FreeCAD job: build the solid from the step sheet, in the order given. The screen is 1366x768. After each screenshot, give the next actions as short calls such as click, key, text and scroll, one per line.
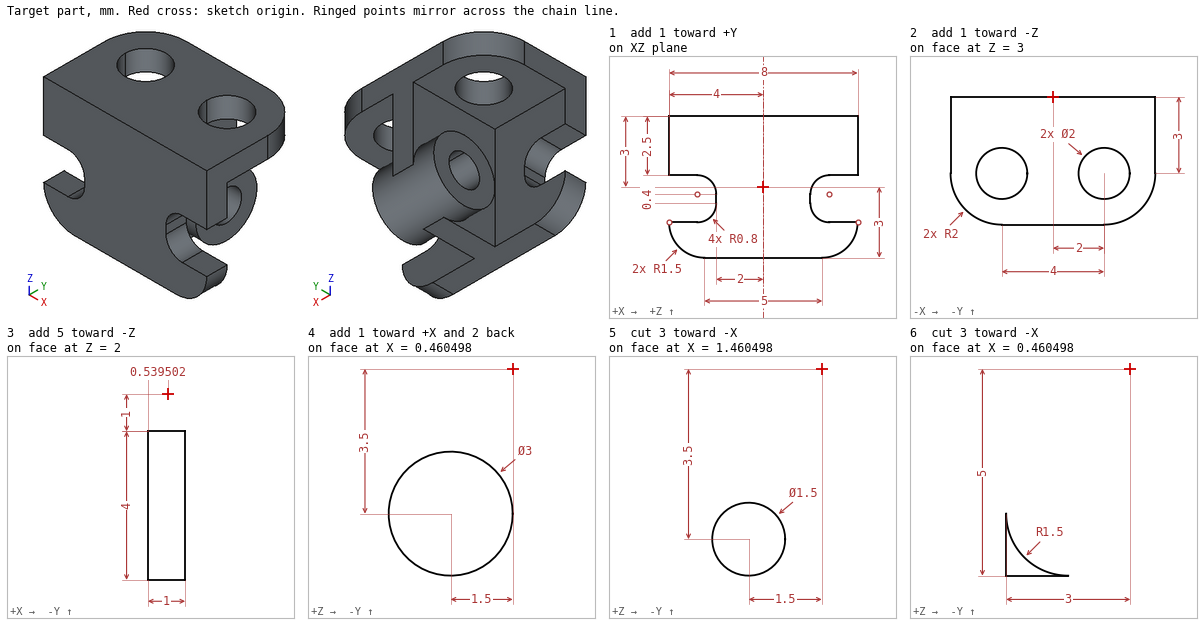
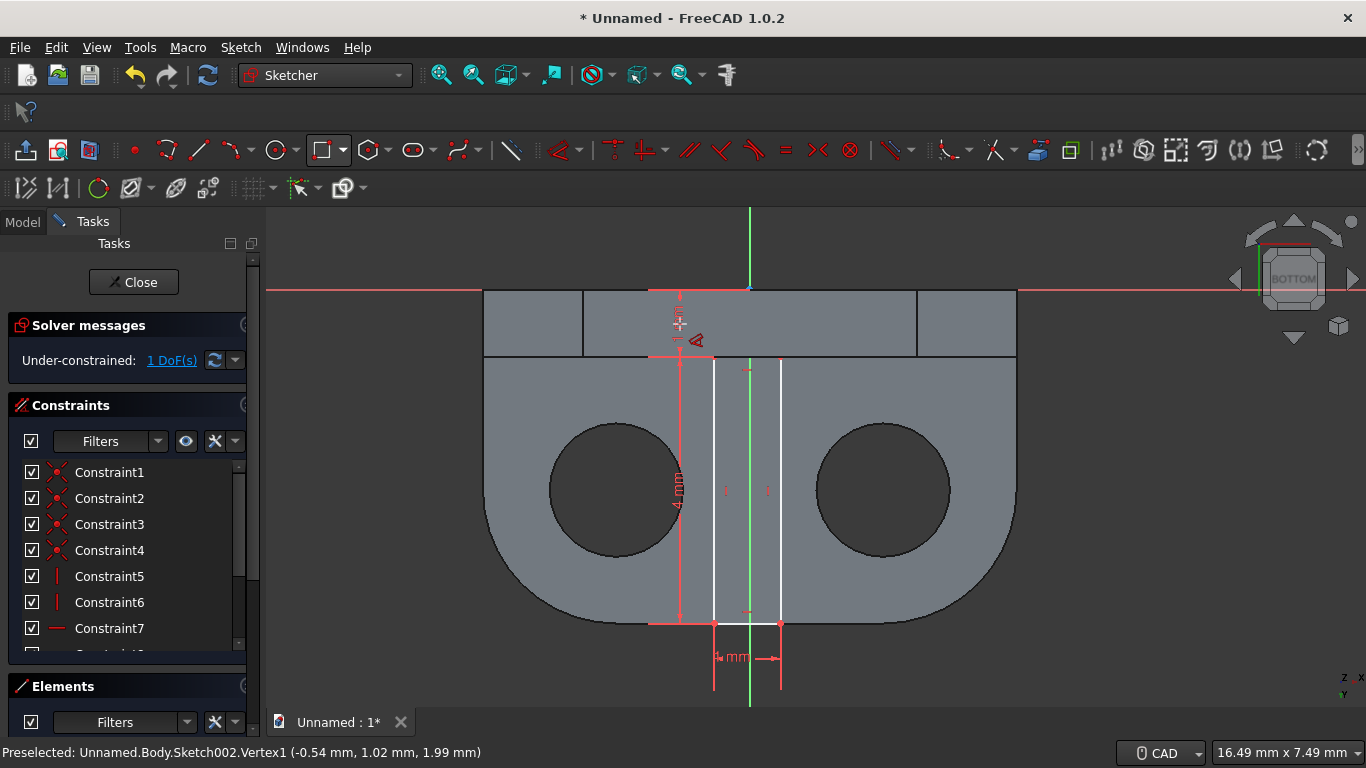
click(714, 357)
click(732, 256)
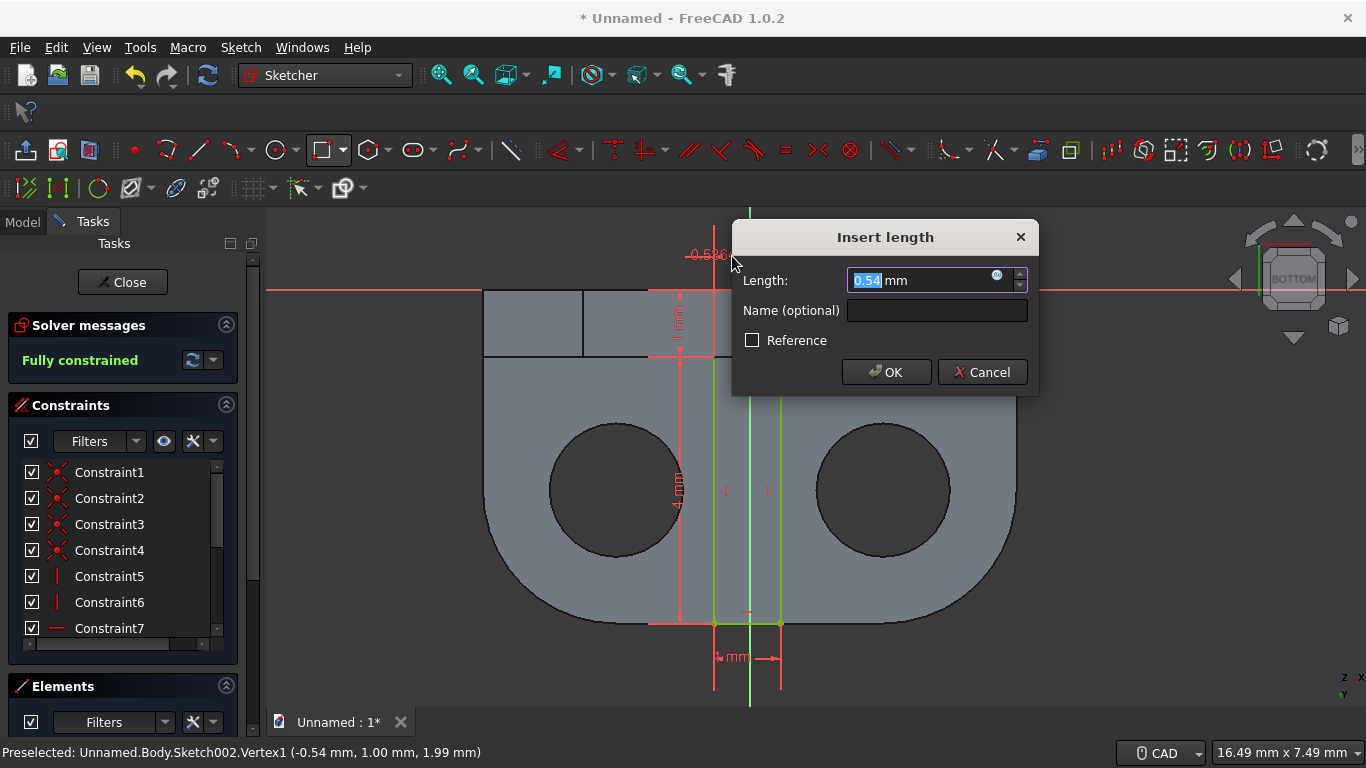
text(0.539502)
key(Return)
key(Escape)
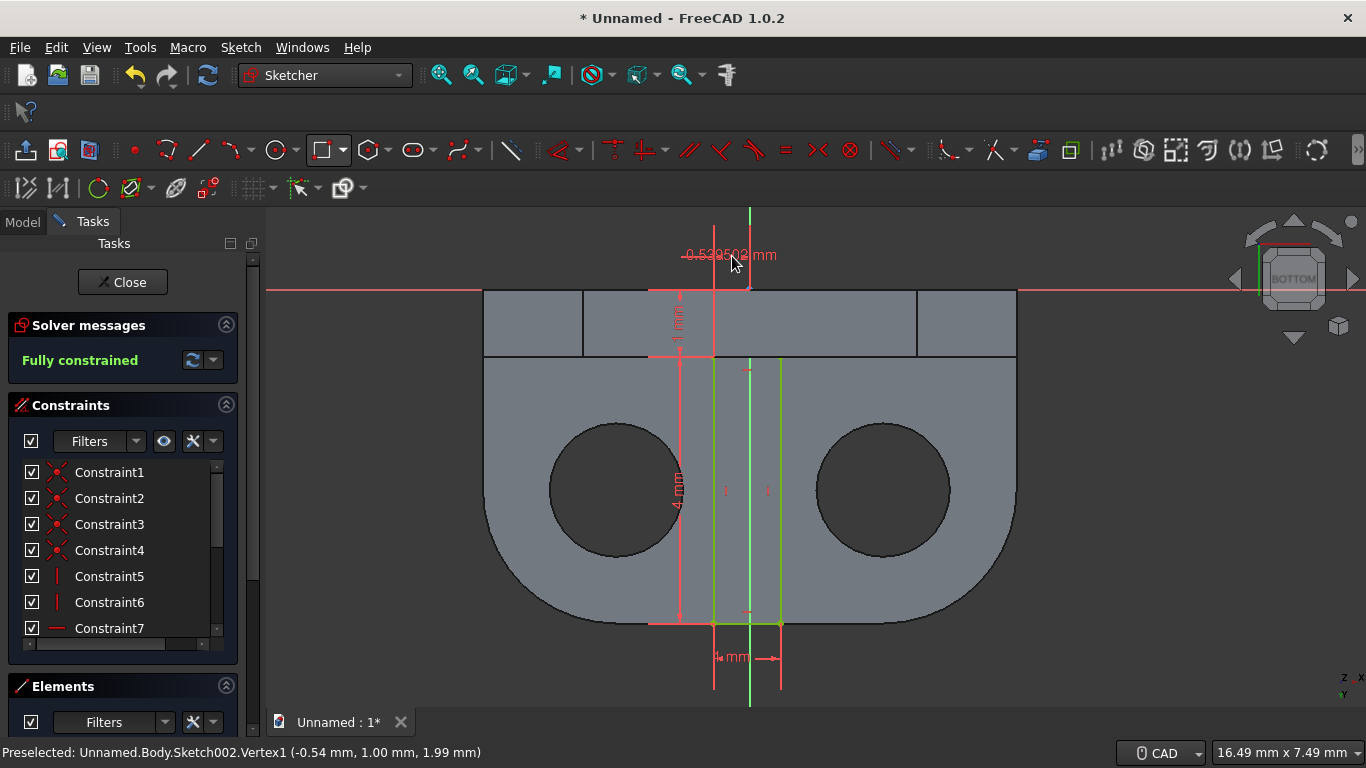
click(123, 282)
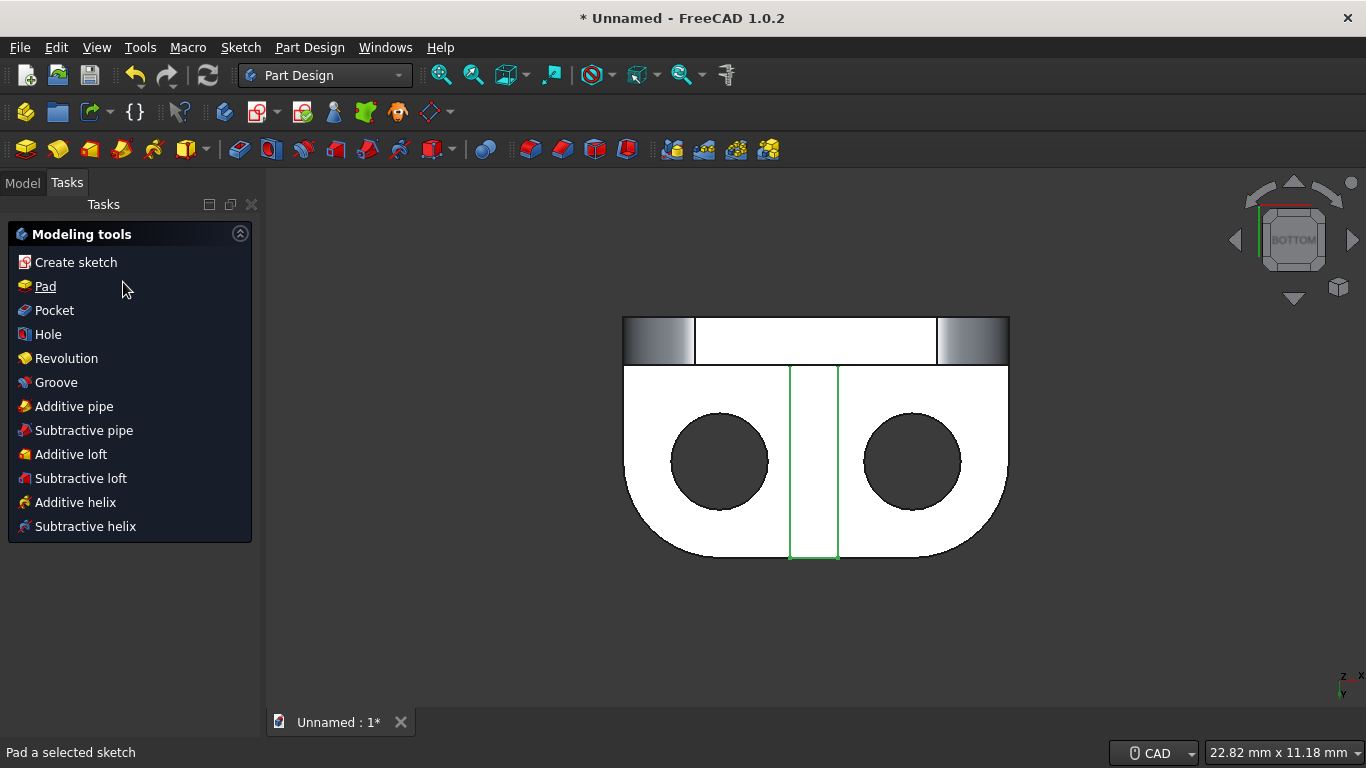
click(26, 150)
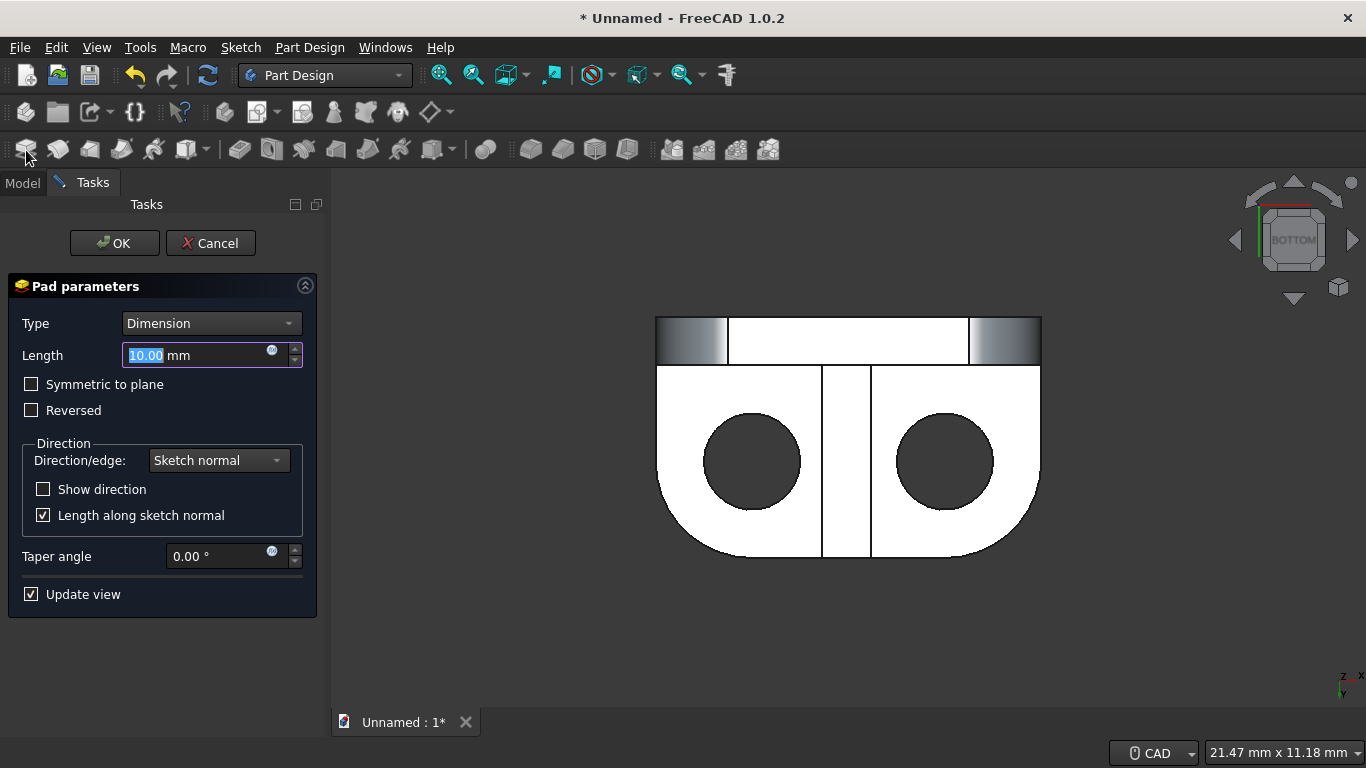
text(5)
key(Tab)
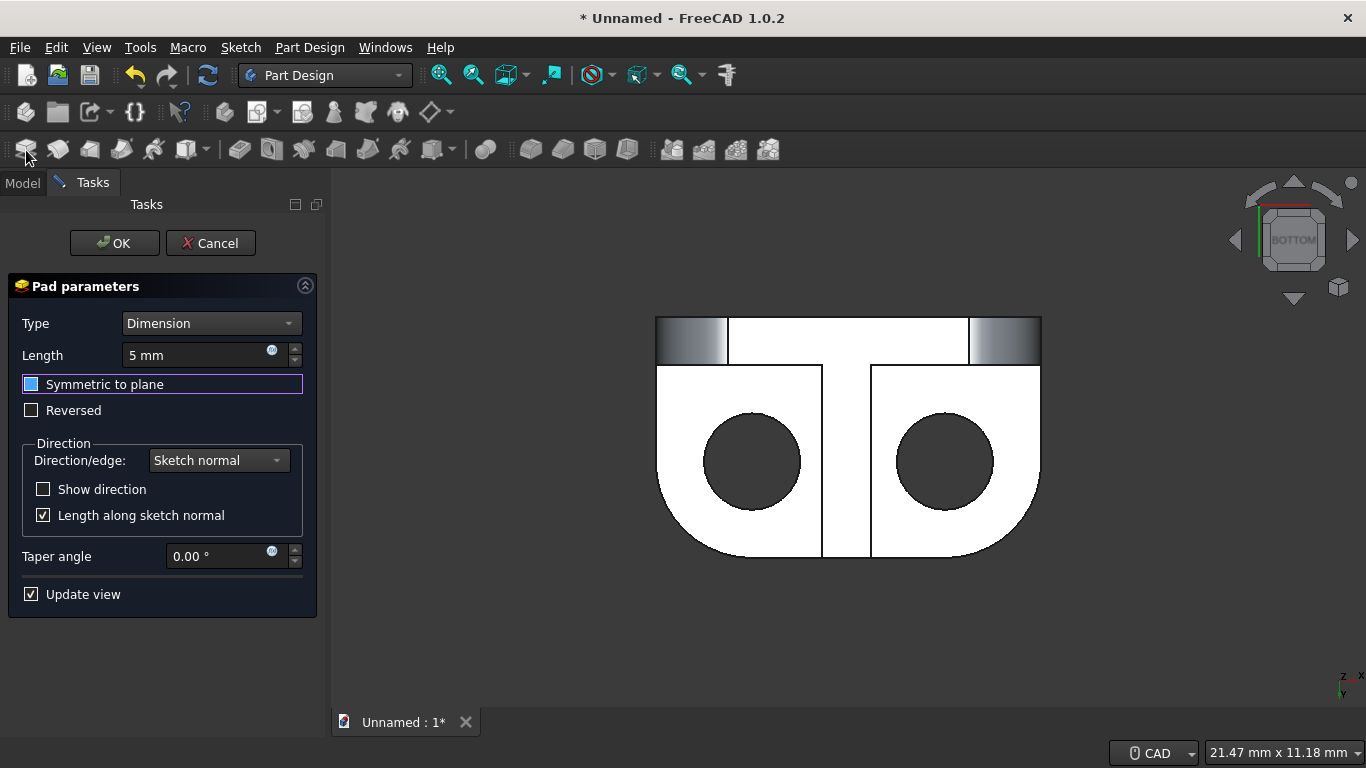
click(115, 243)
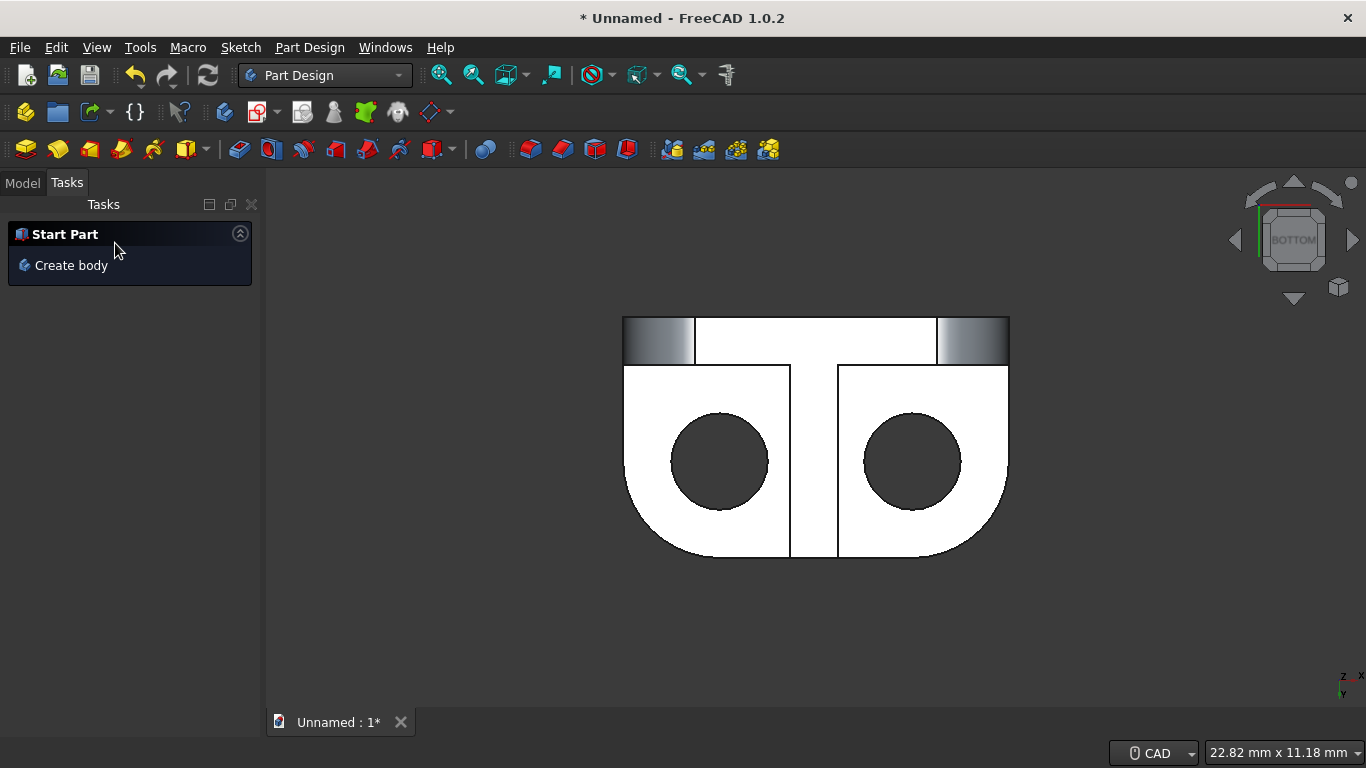
click(442, 76)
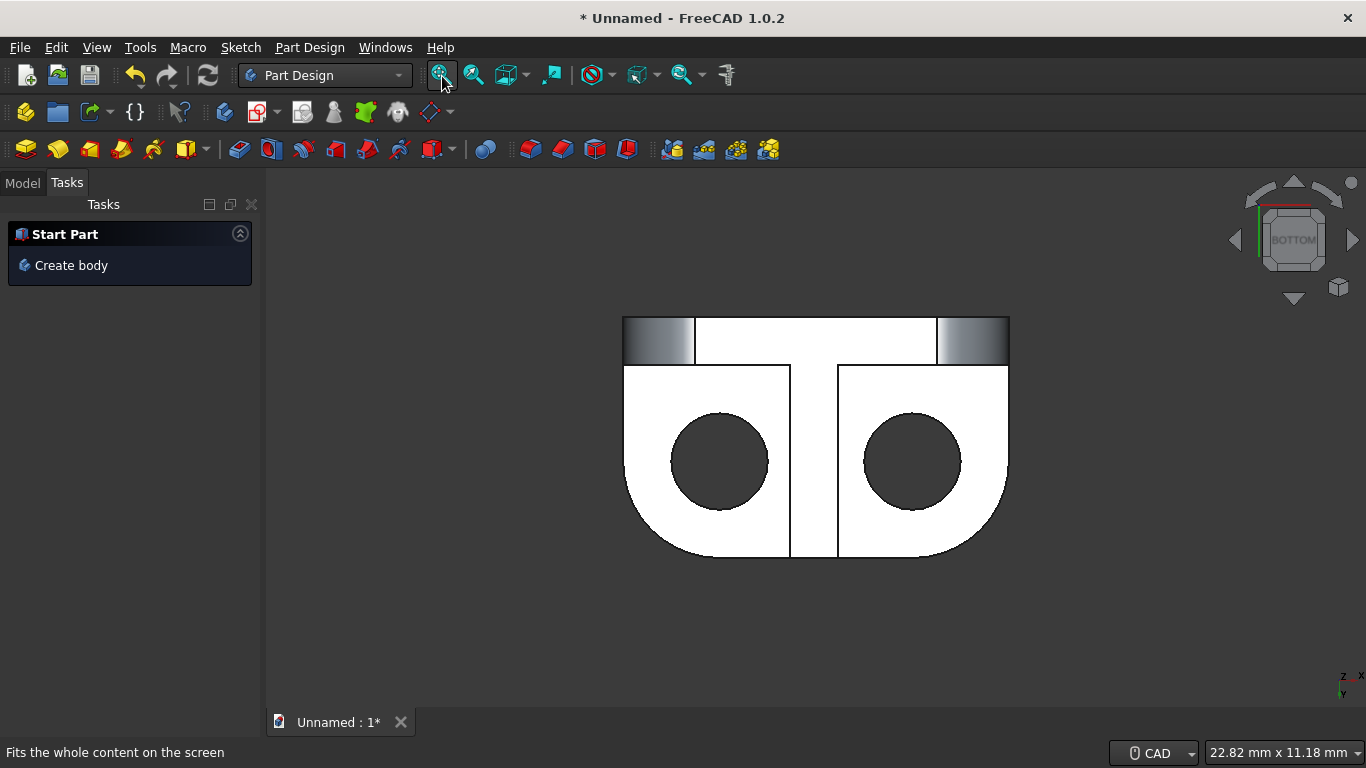
key(0)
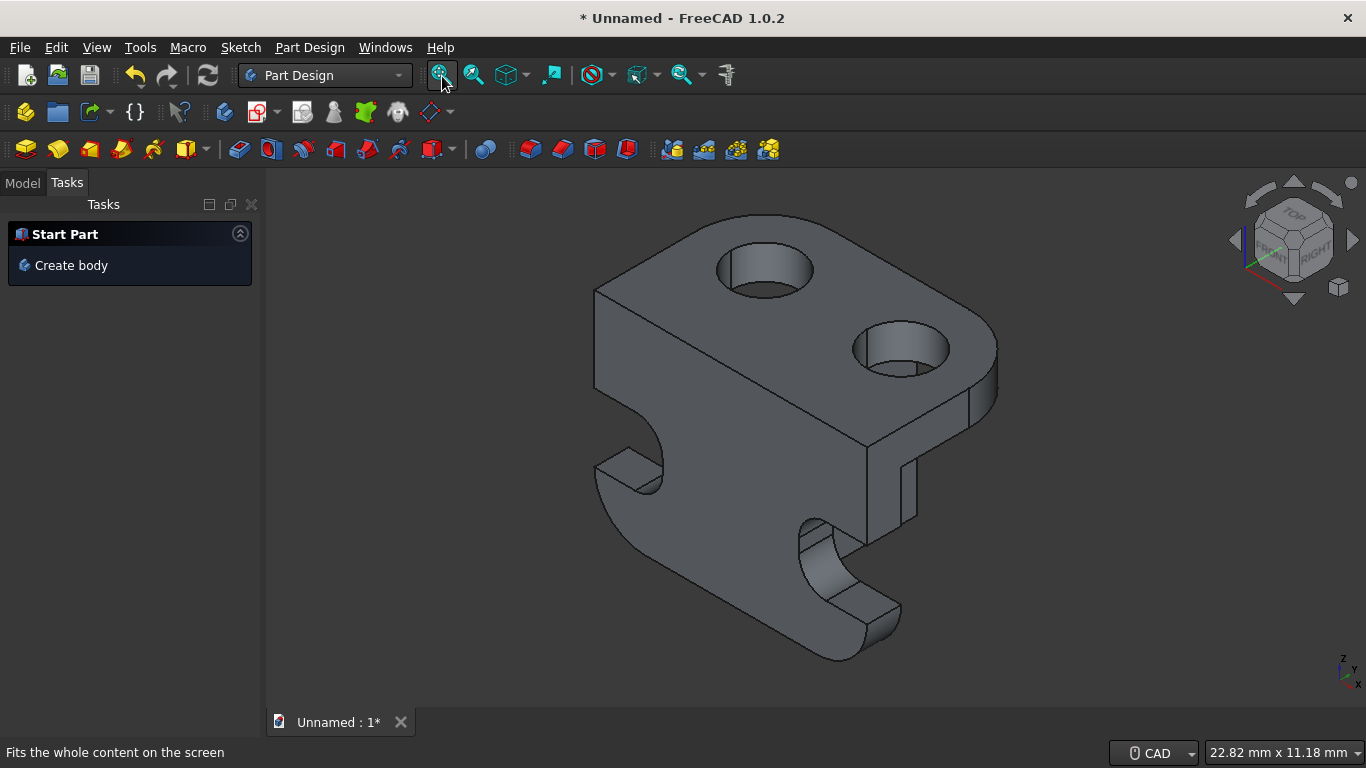
key(3)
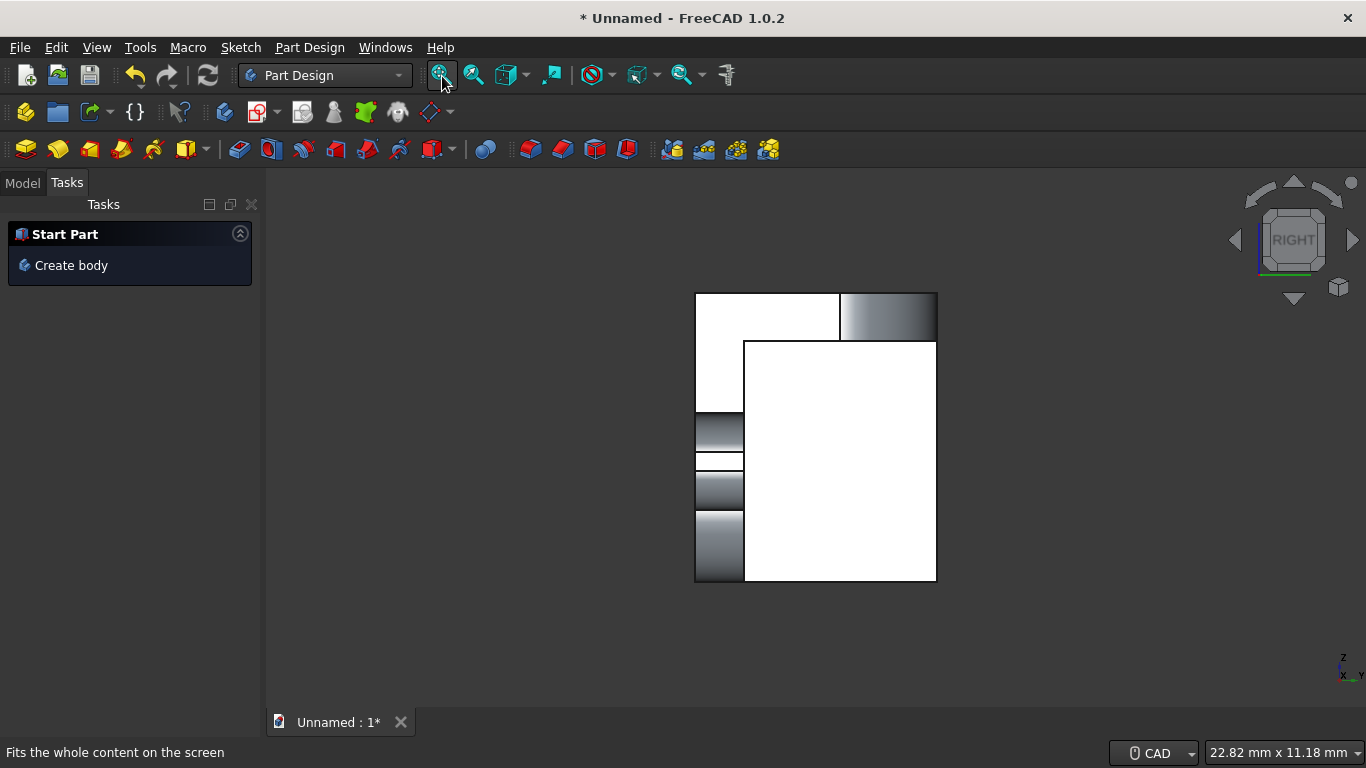
click(840, 461)